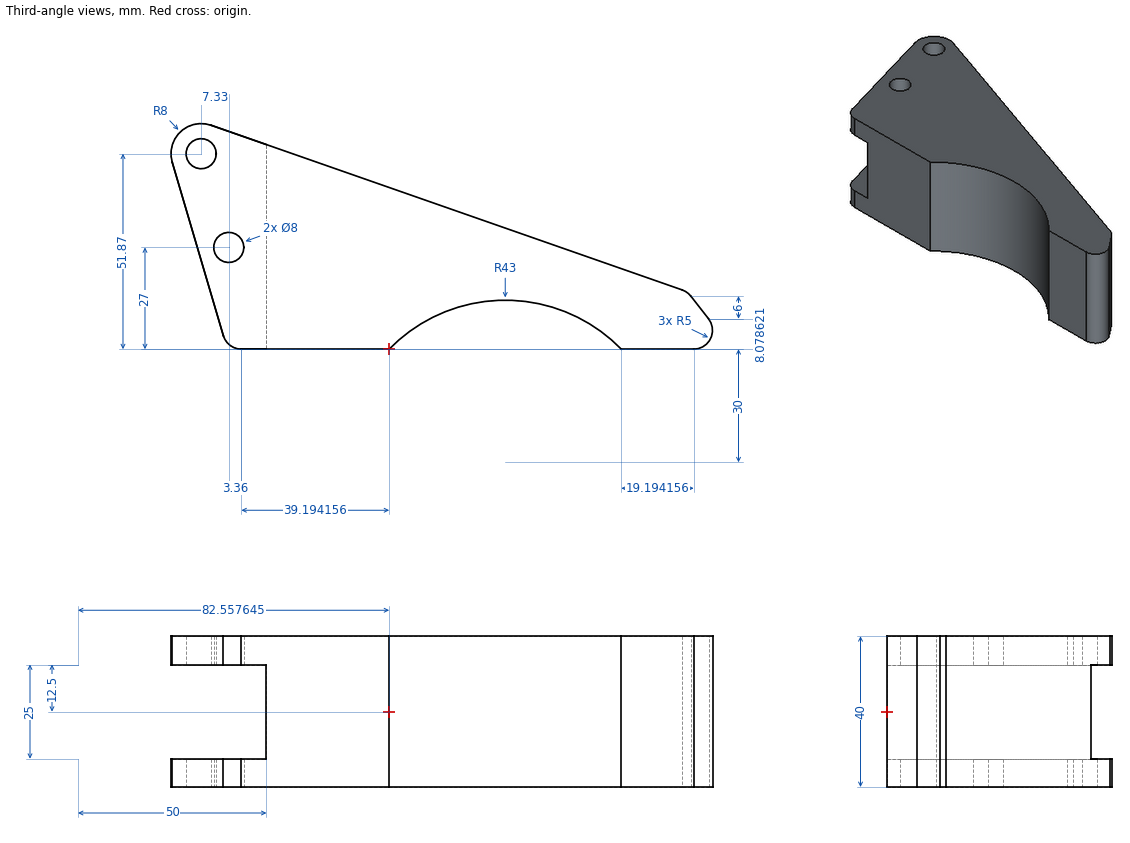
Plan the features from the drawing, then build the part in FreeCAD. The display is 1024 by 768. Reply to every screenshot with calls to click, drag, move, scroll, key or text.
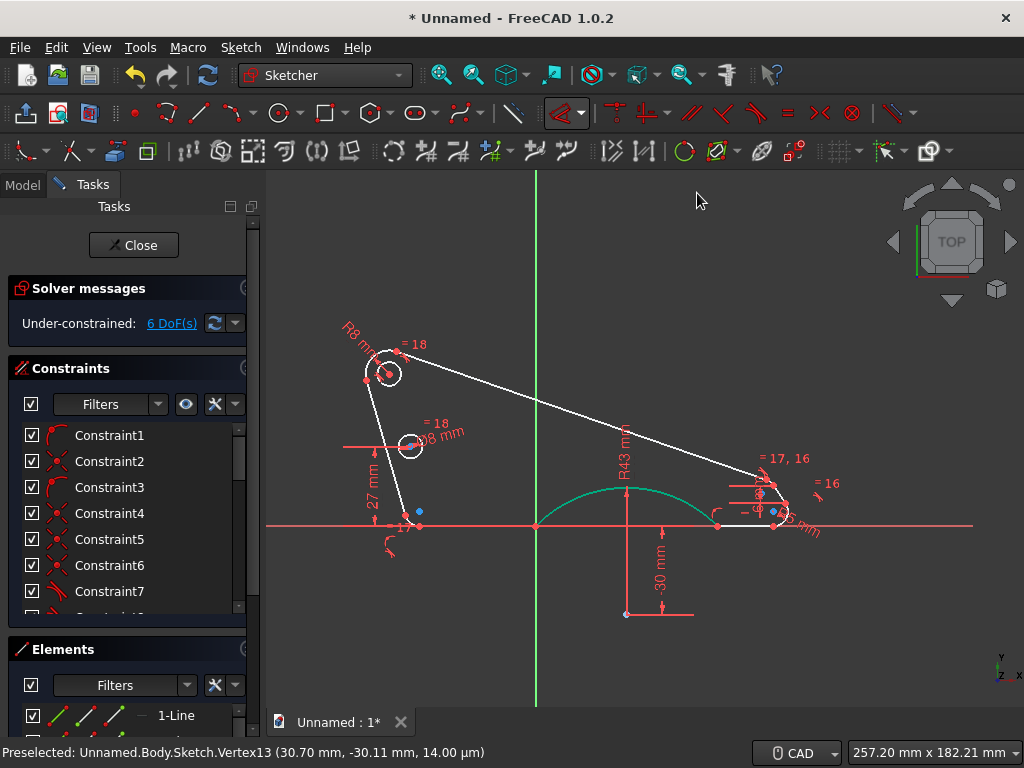
click(389, 374)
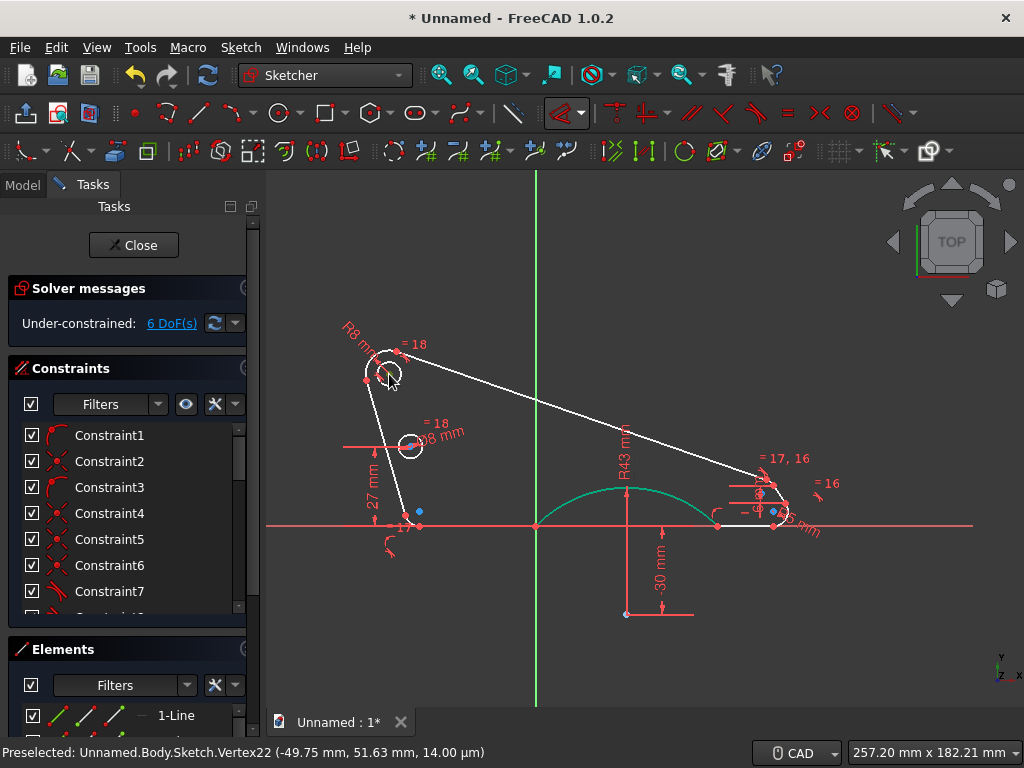
key(i)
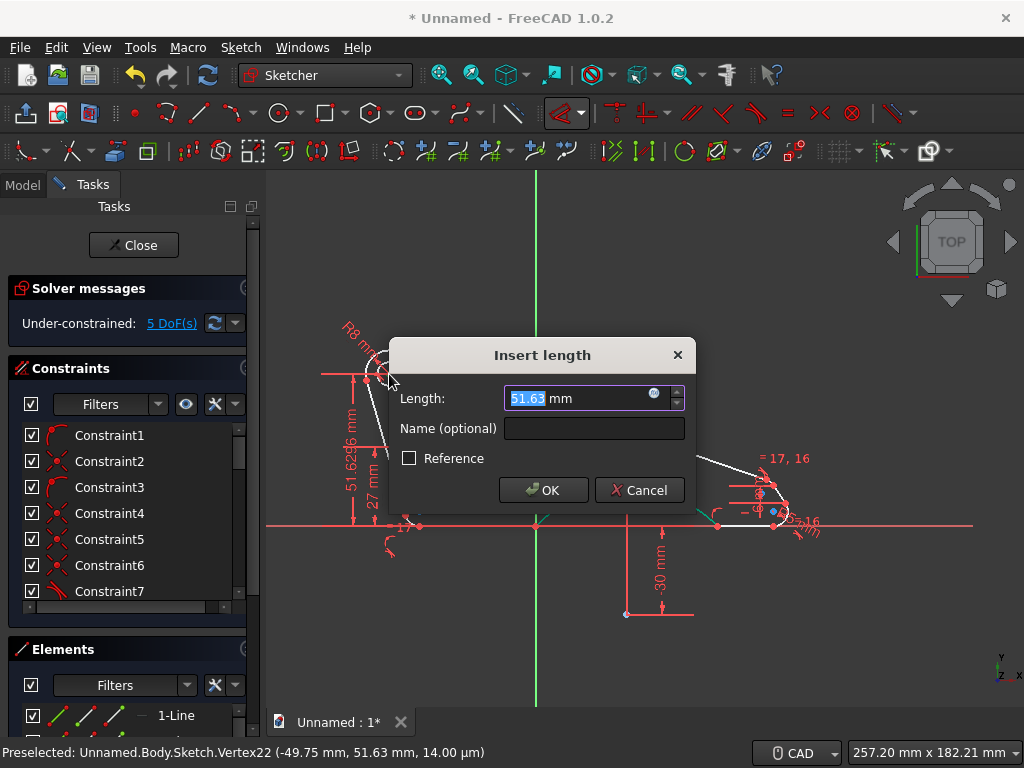
text(51.87)
key(Return)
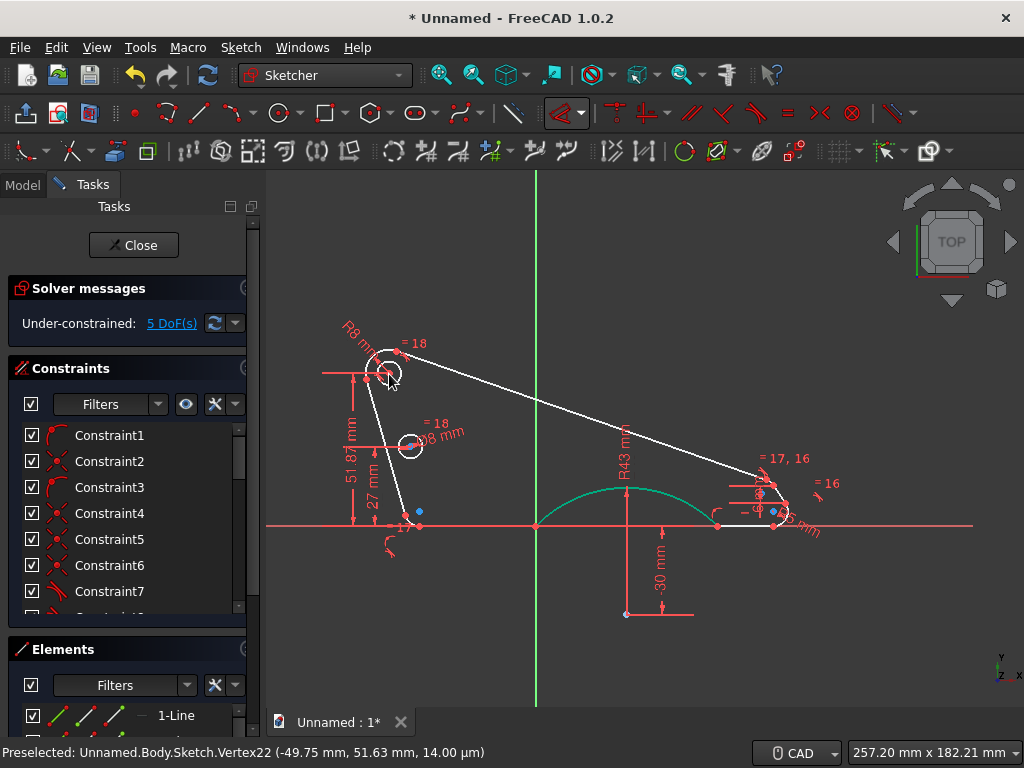
scroll(420, 526, up, 7)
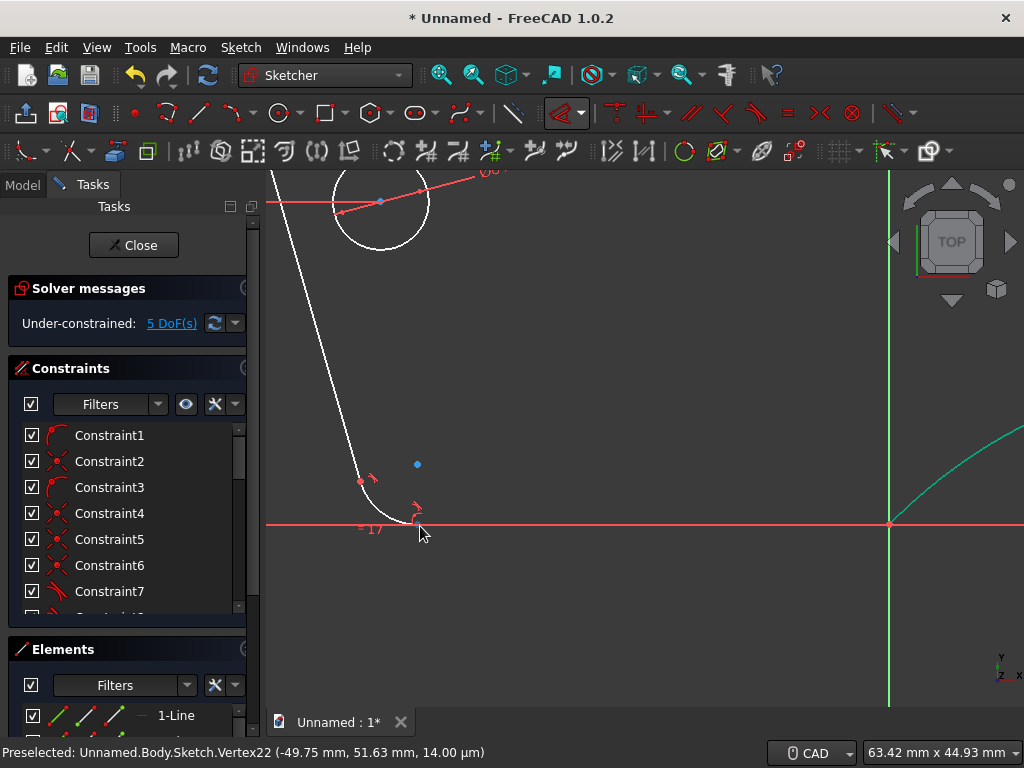
click(418, 525)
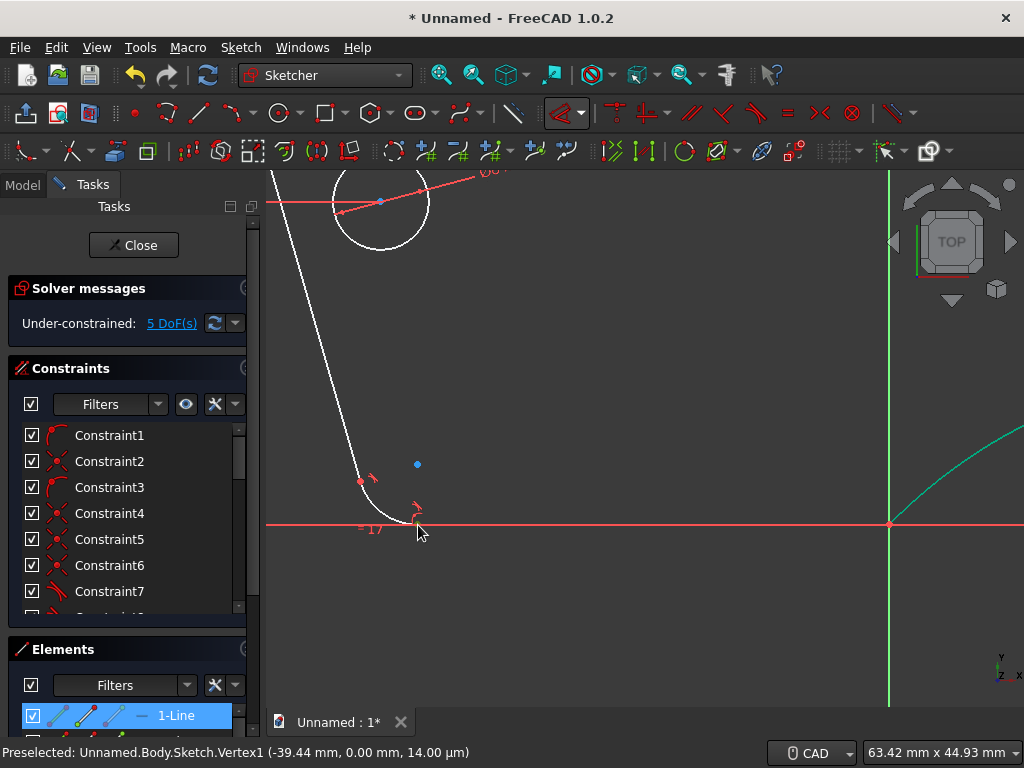
click(381, 202)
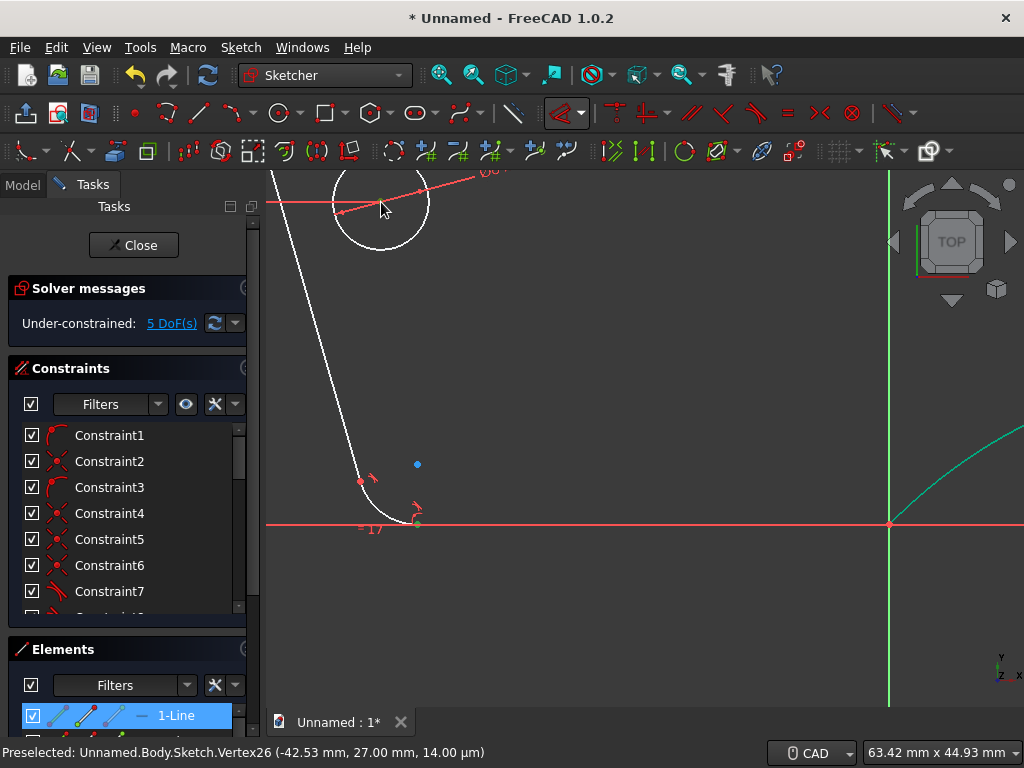
click(584, 114)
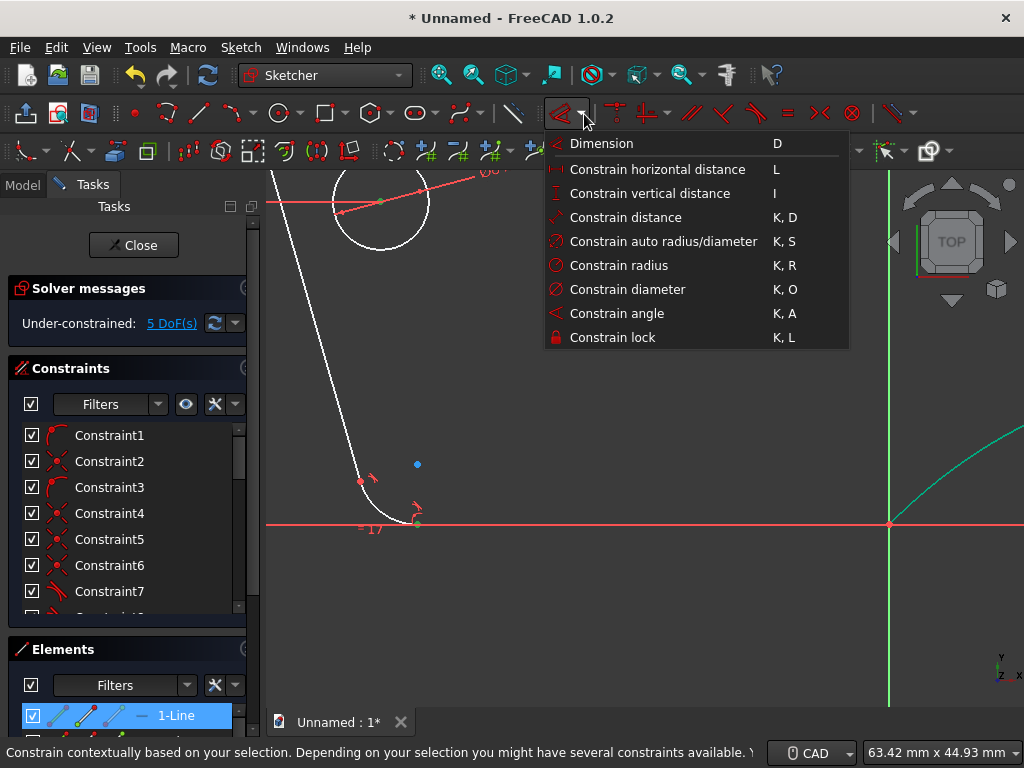
click(697, 169)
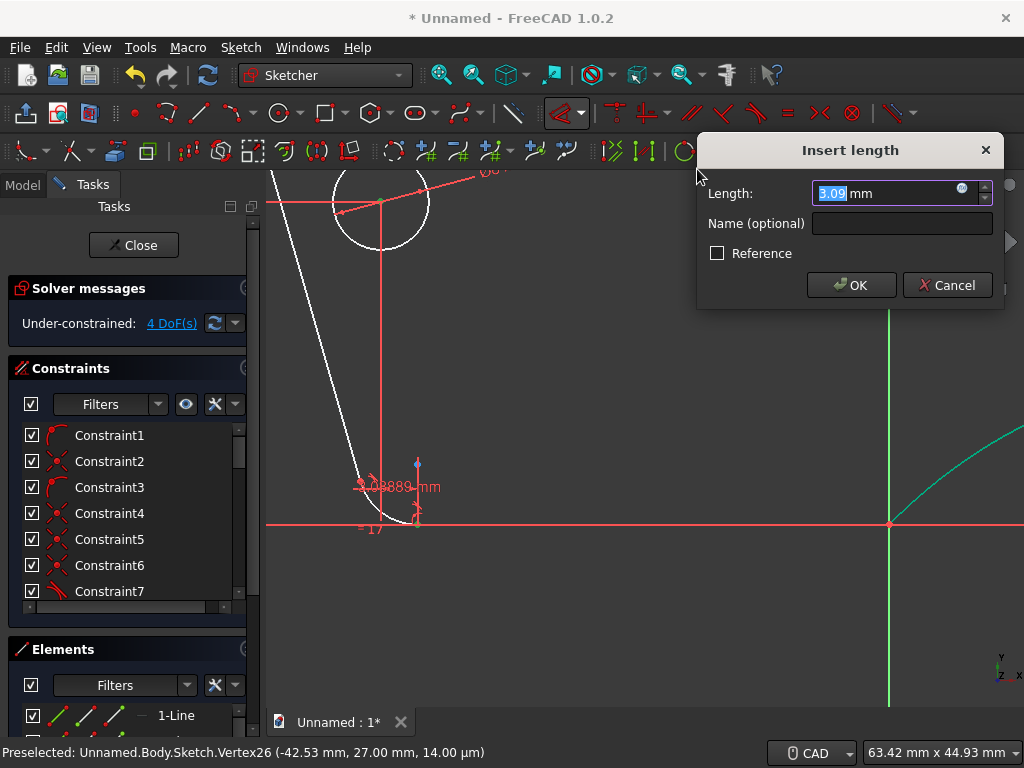
text(3.36)
key(Return)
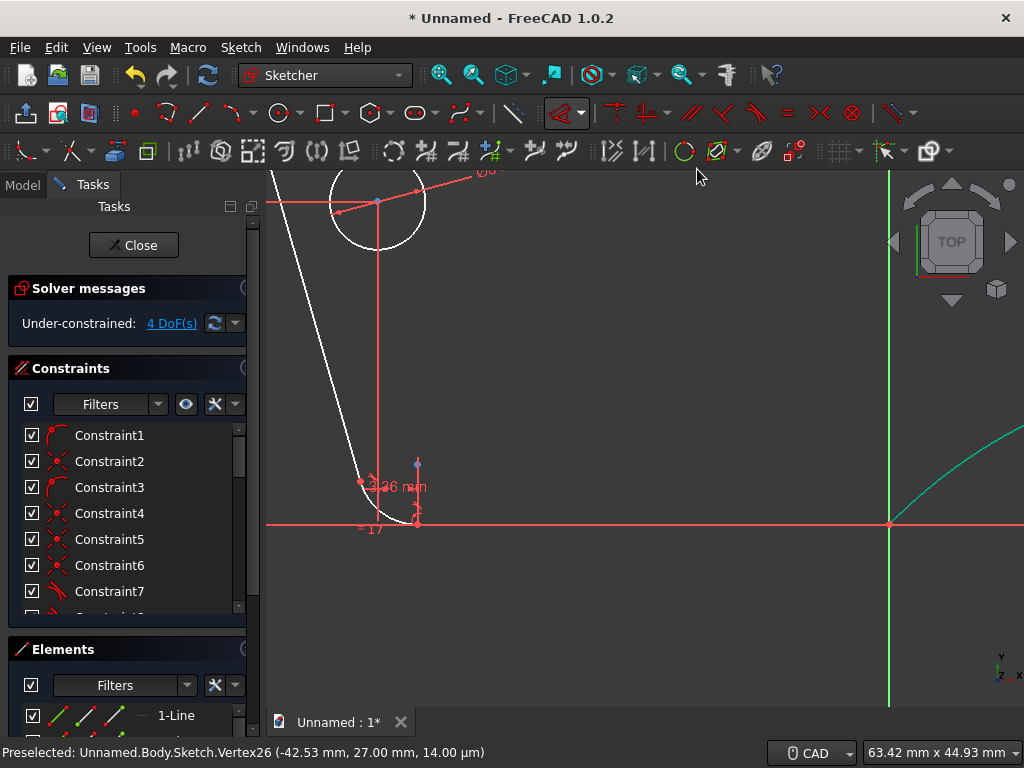
click(378, 202)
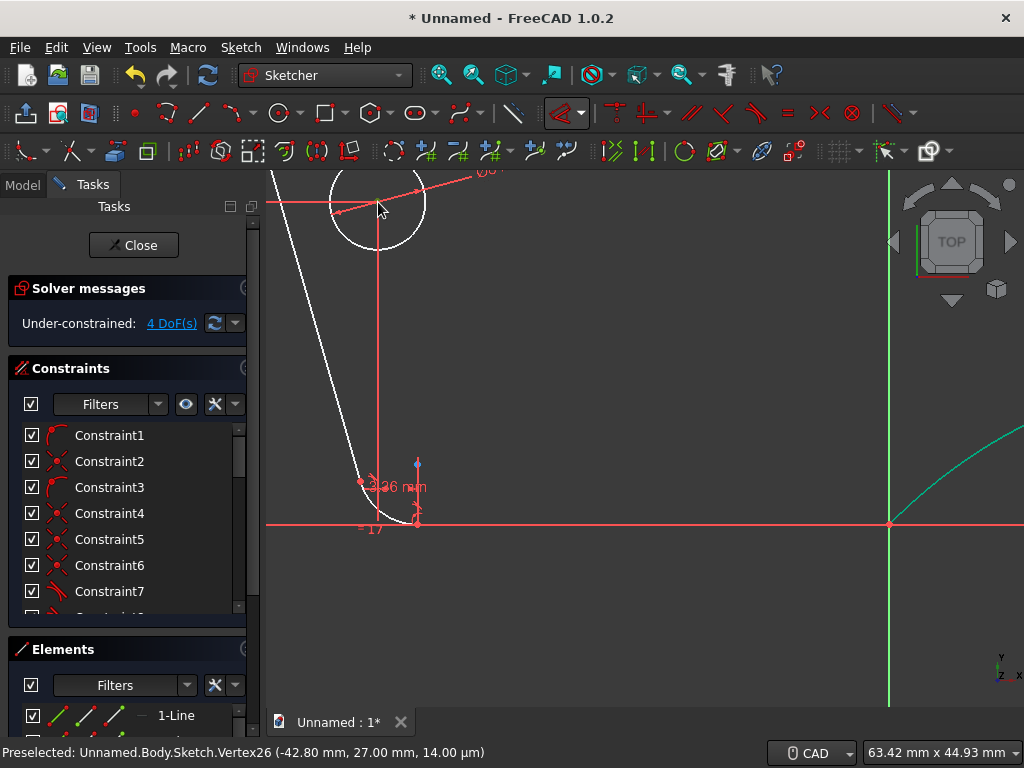
scroll(420, 527, down, 7)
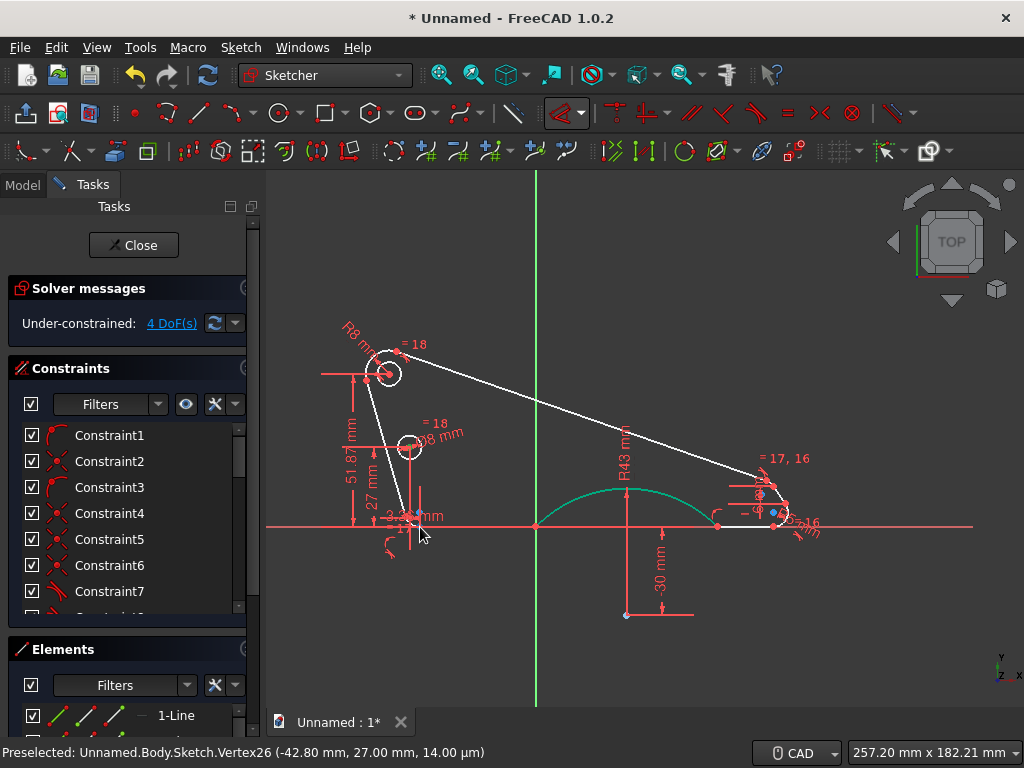
scroll(389, 374, up, 4)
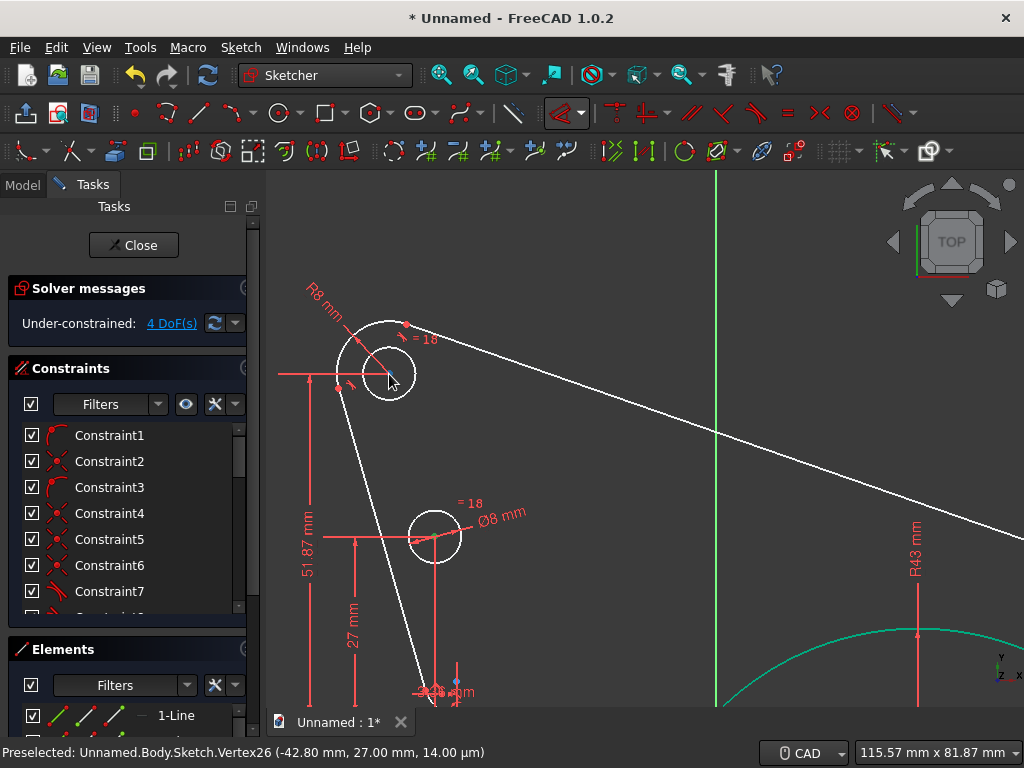
click(389, 374)